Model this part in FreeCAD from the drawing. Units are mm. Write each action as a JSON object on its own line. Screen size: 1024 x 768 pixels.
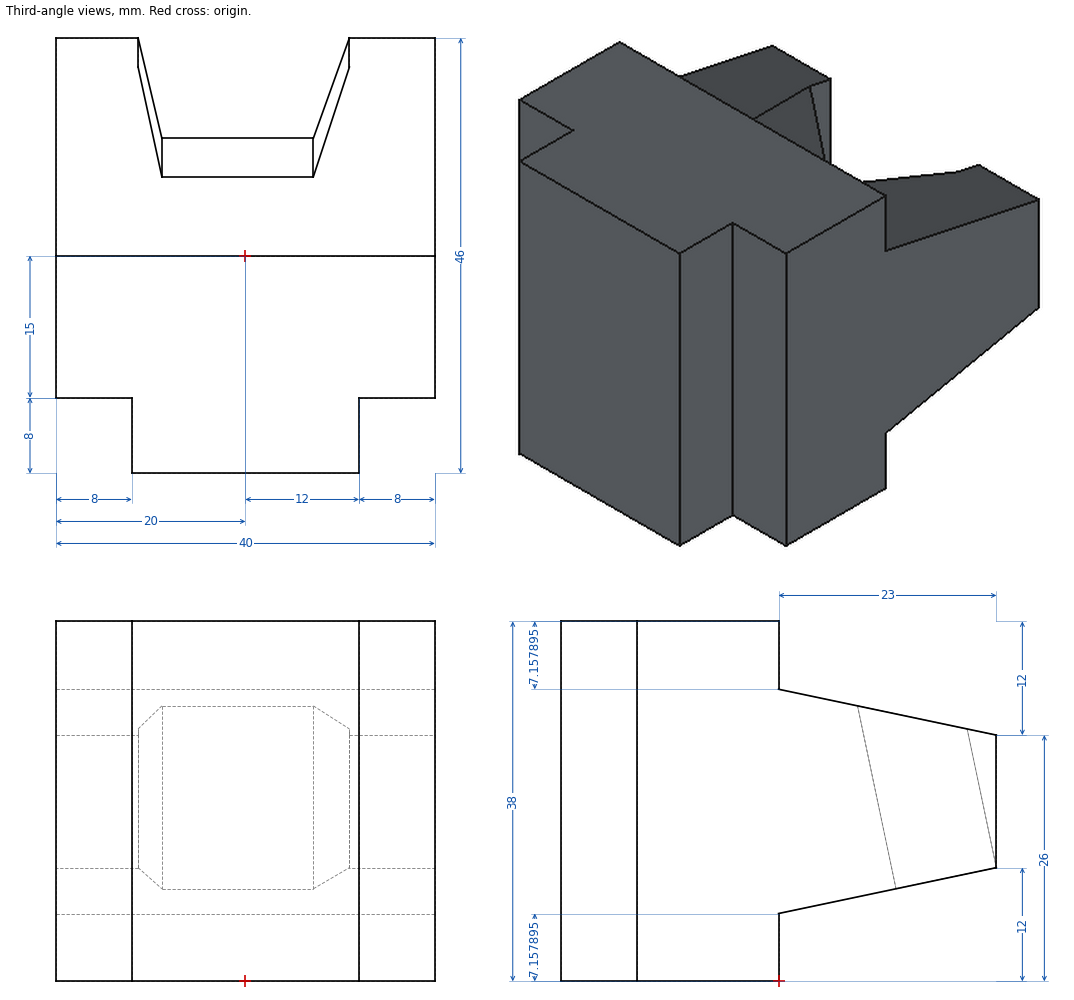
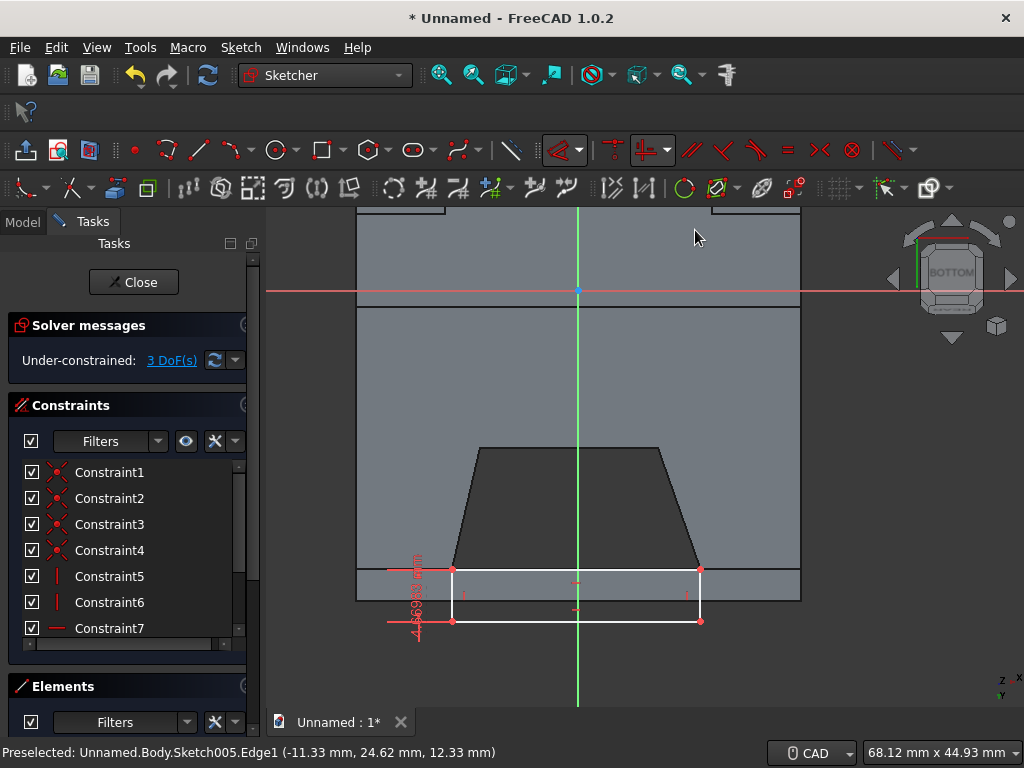
{"action": "left_click", "coordinate": [526, 622]}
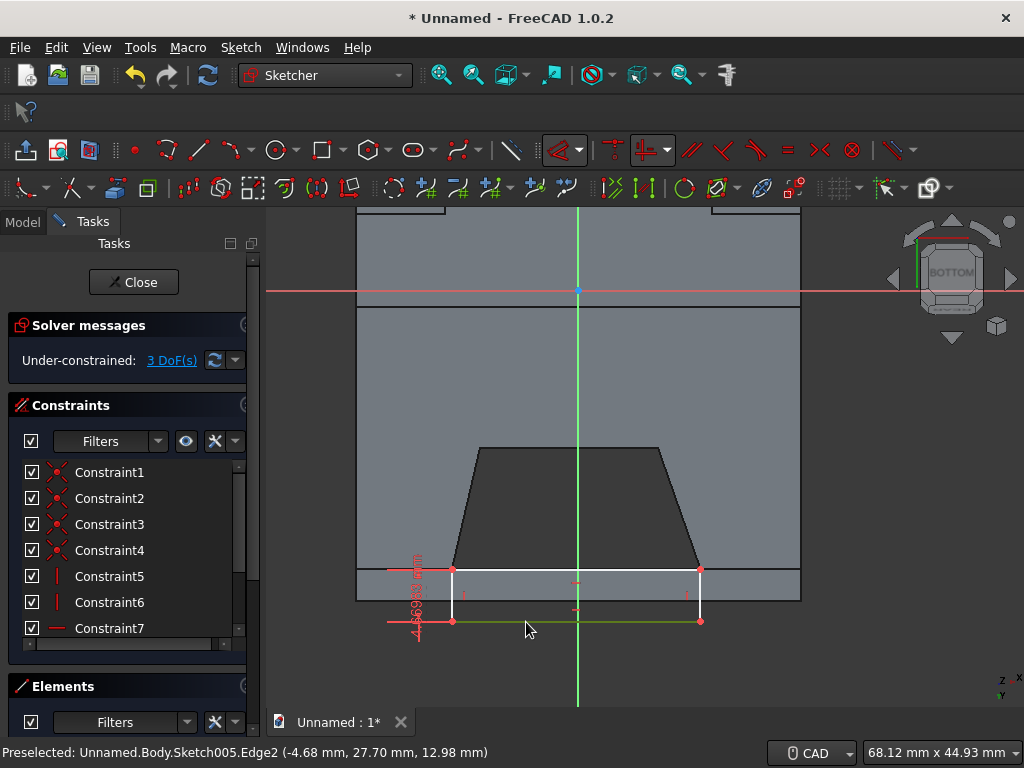
{"action": "key", "text": "l"}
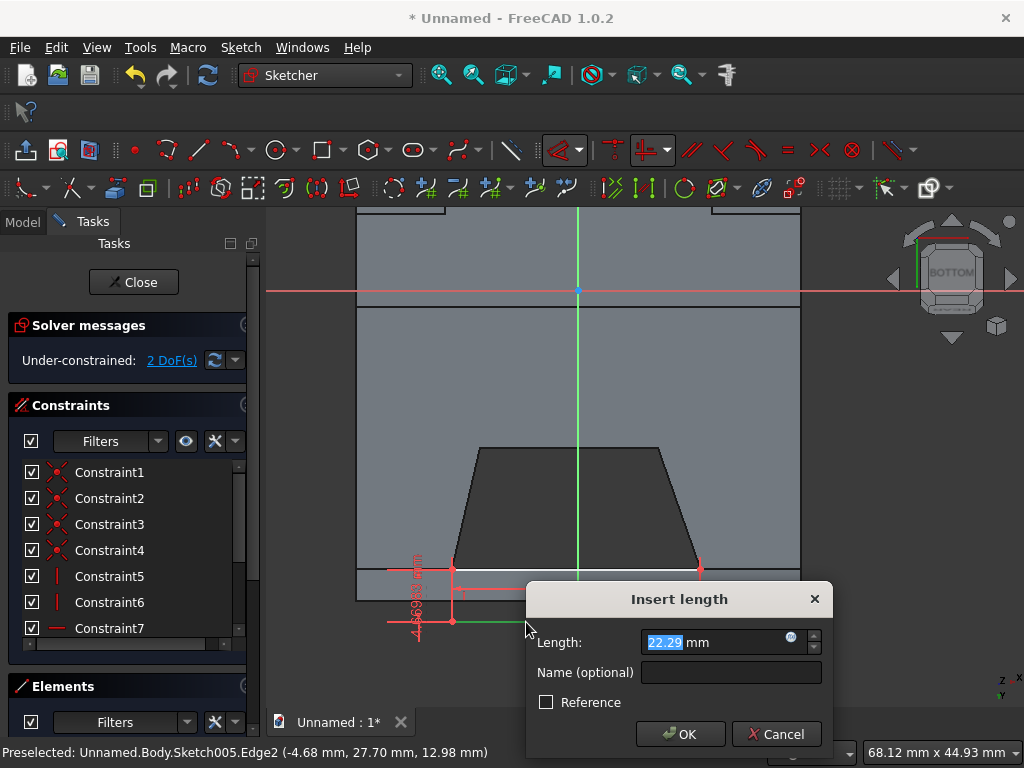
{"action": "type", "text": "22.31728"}
{"action": "key", "text": "Return"}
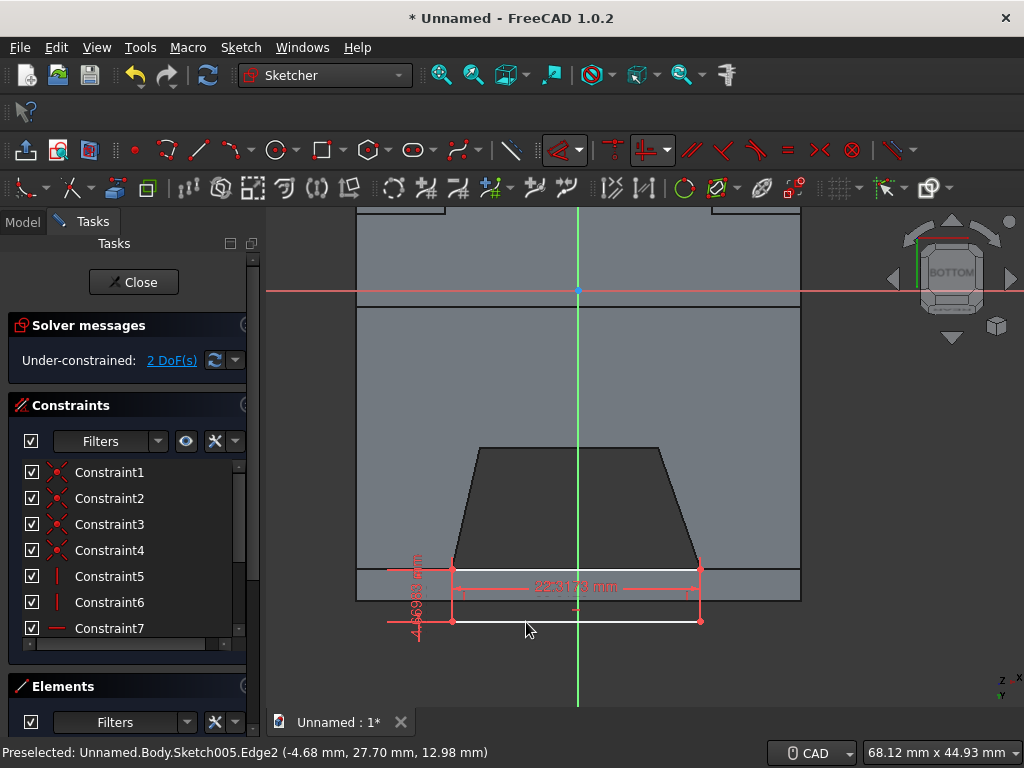
{"action": "left_click", "coordinate": [452, 570]}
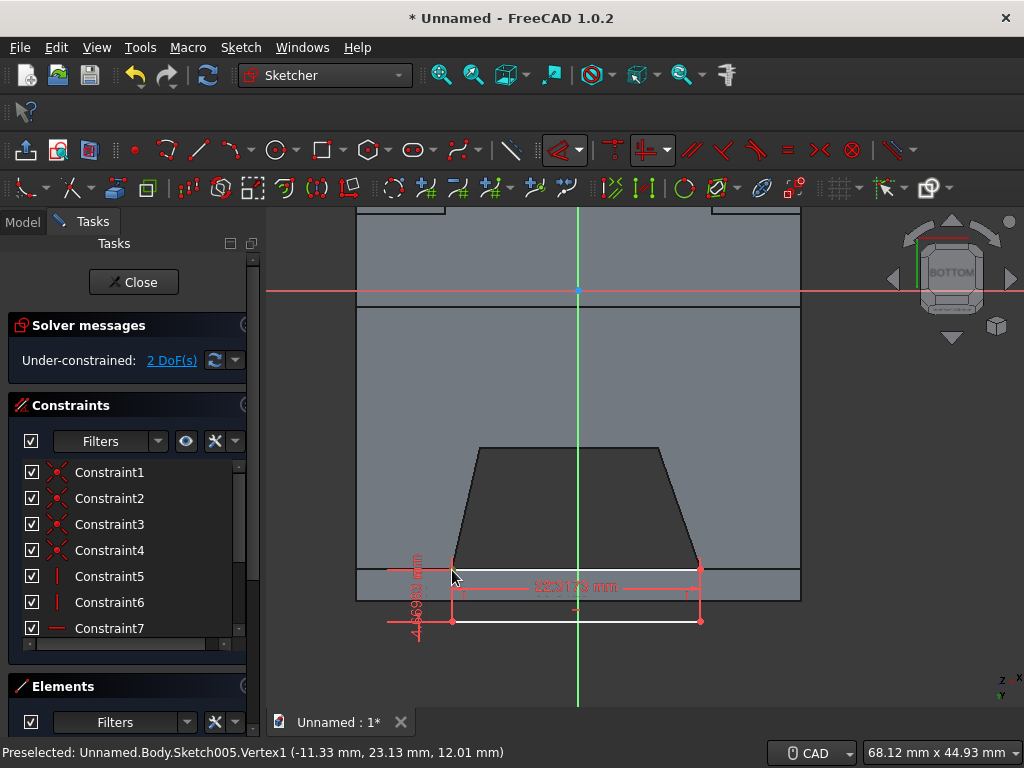
{"action": "left_click", "coordinate": [582, 150]}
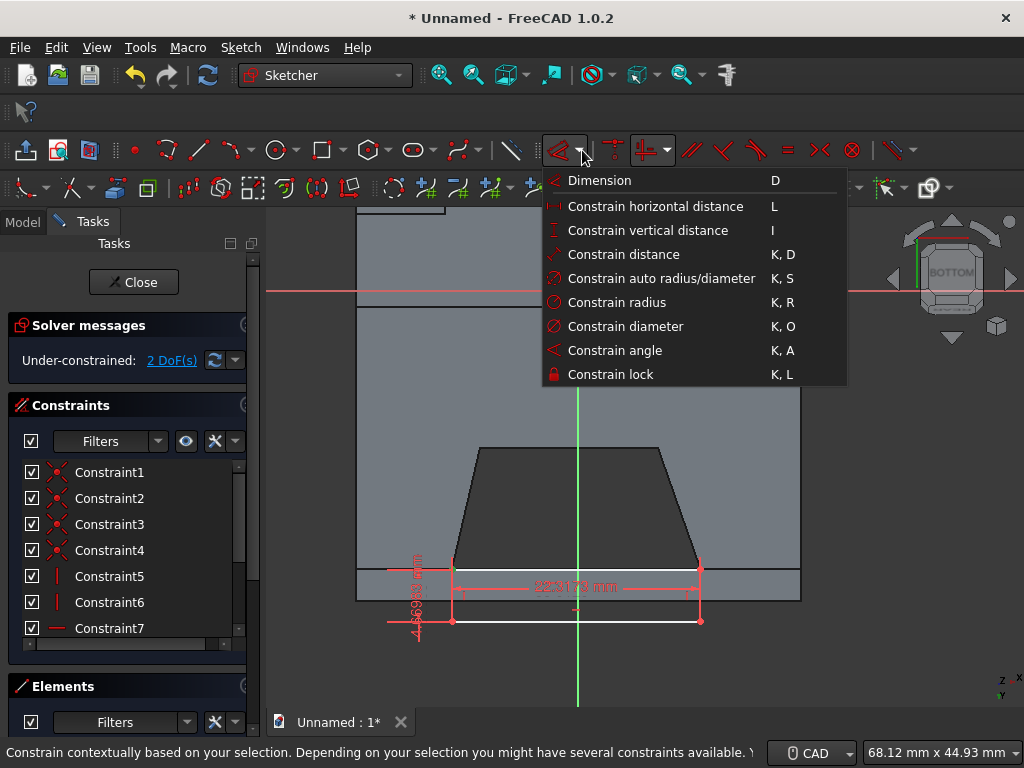
{"action": "left_click", "coordinate": [695, 206]}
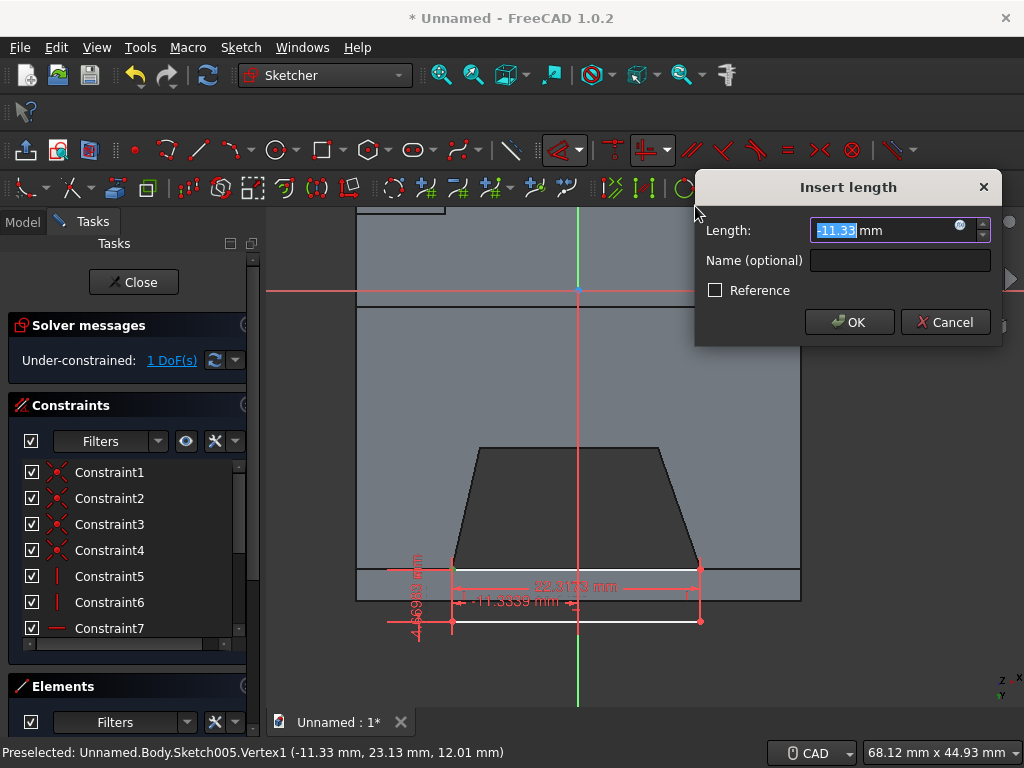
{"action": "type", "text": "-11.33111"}
{"action": "key", "text": "Return"}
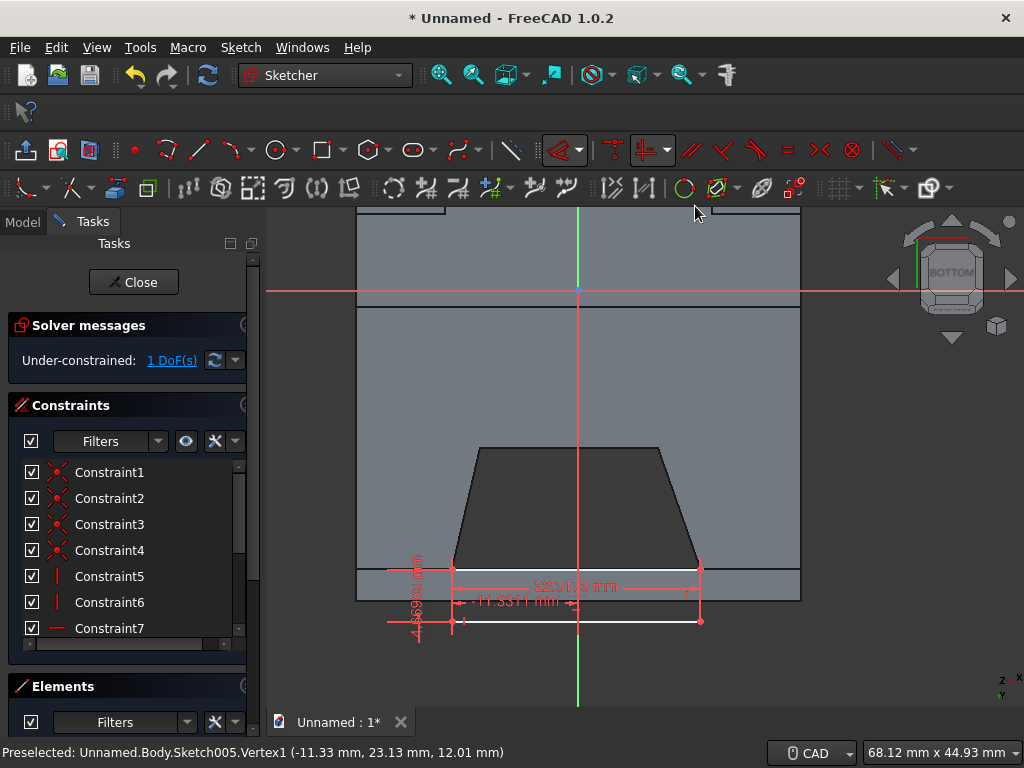
{"action": "left_click", "coordinate": [452, 570]}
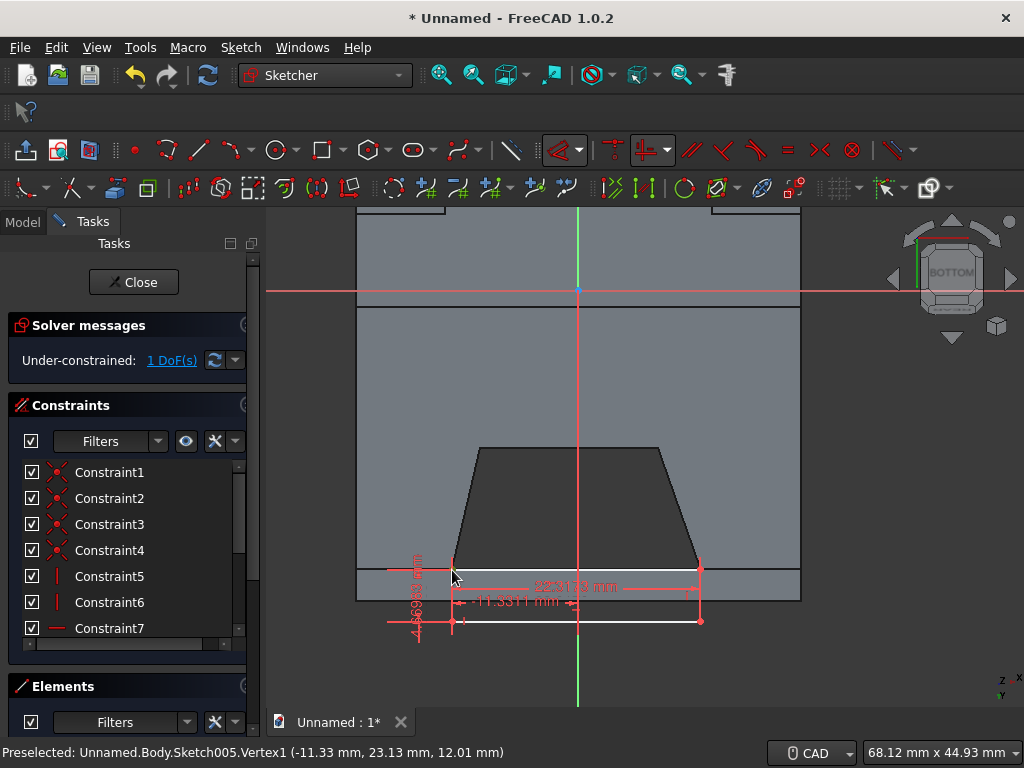
{"action": "left_click", "coordinate": [582, 150]}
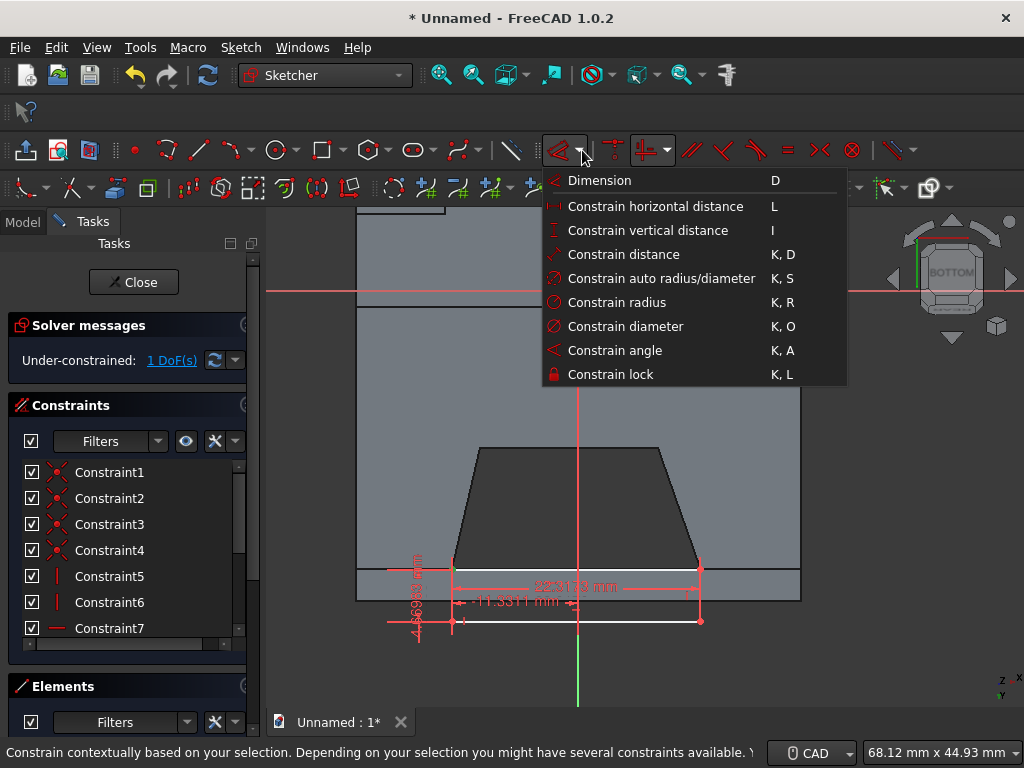
{"action": "left_click", "coordinate": [695, 230]}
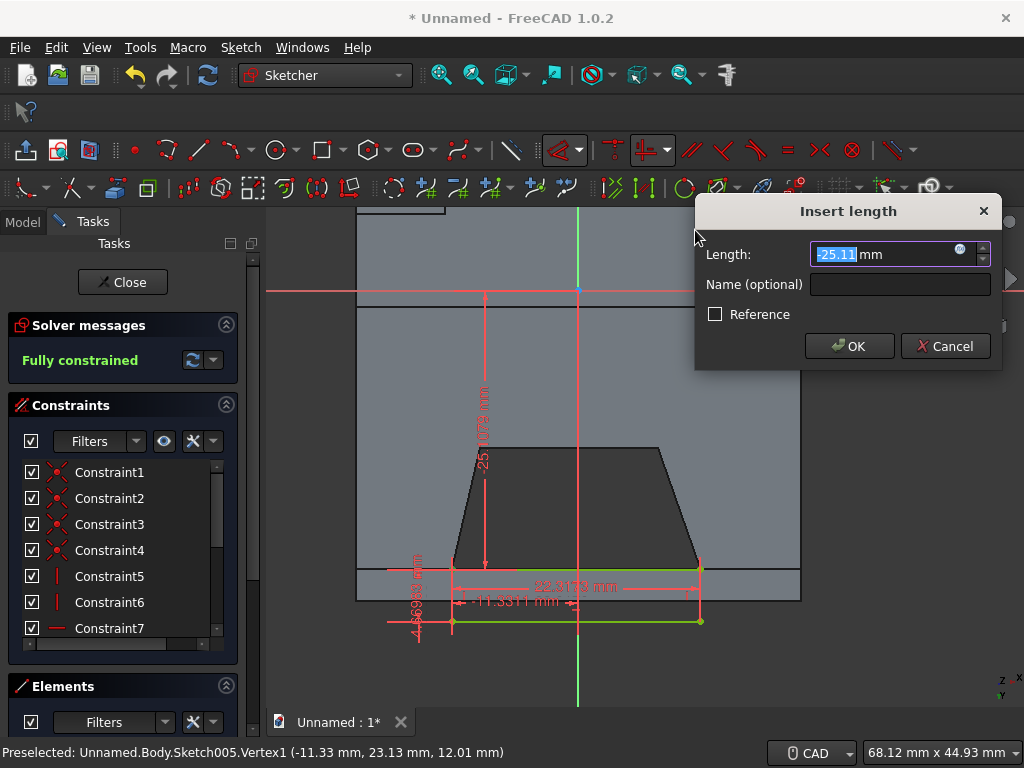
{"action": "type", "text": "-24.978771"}
{"action": "key", "text": "Return"}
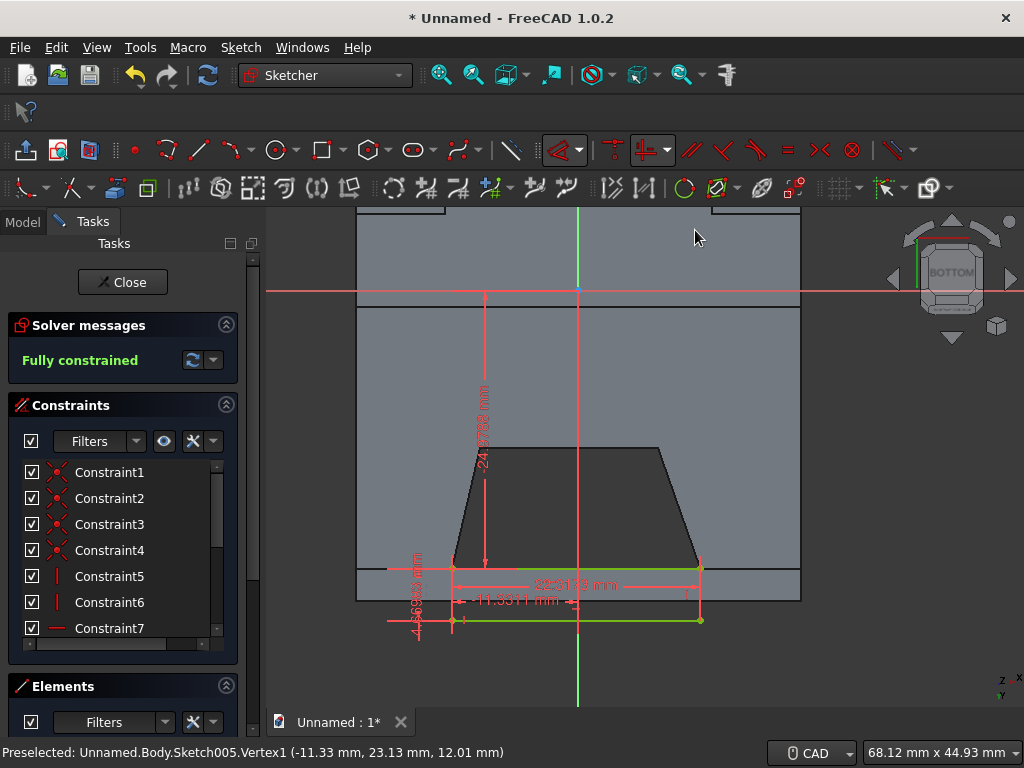
{"action": "left_click", "coordinate": [123, 282]}